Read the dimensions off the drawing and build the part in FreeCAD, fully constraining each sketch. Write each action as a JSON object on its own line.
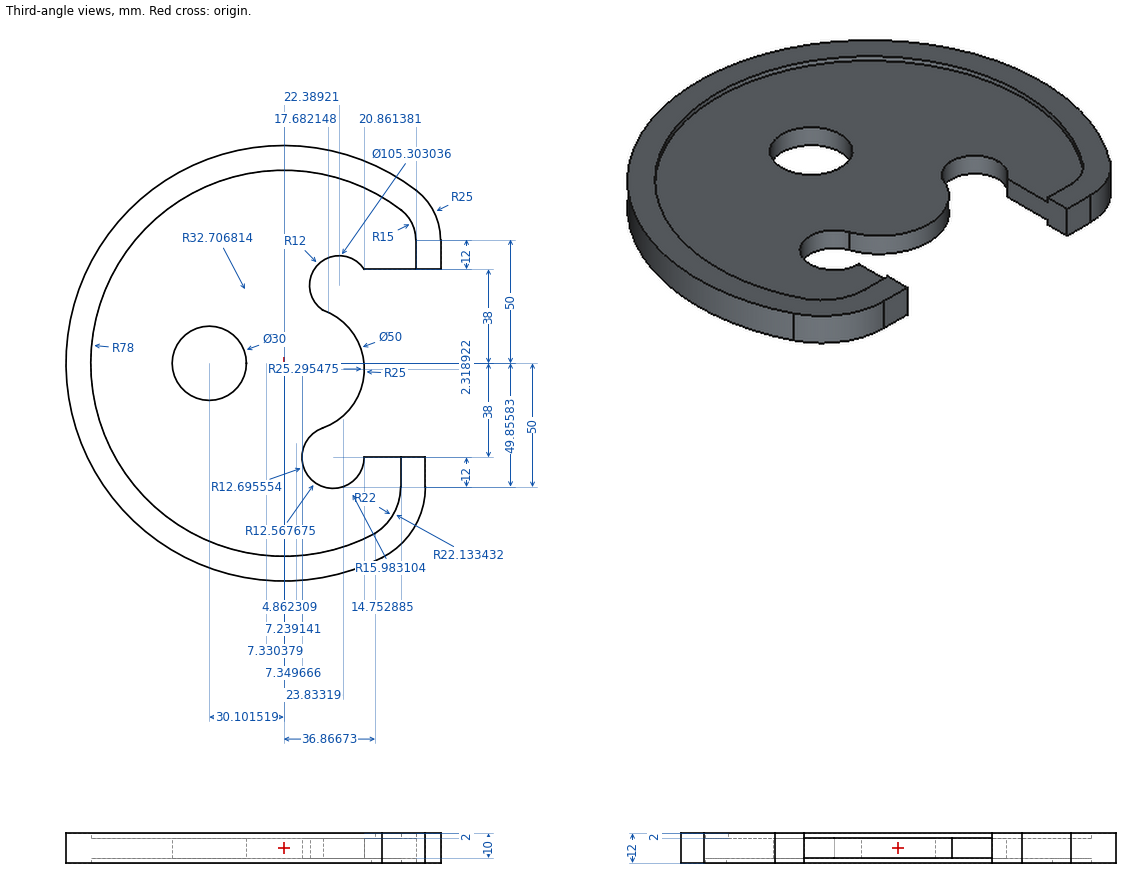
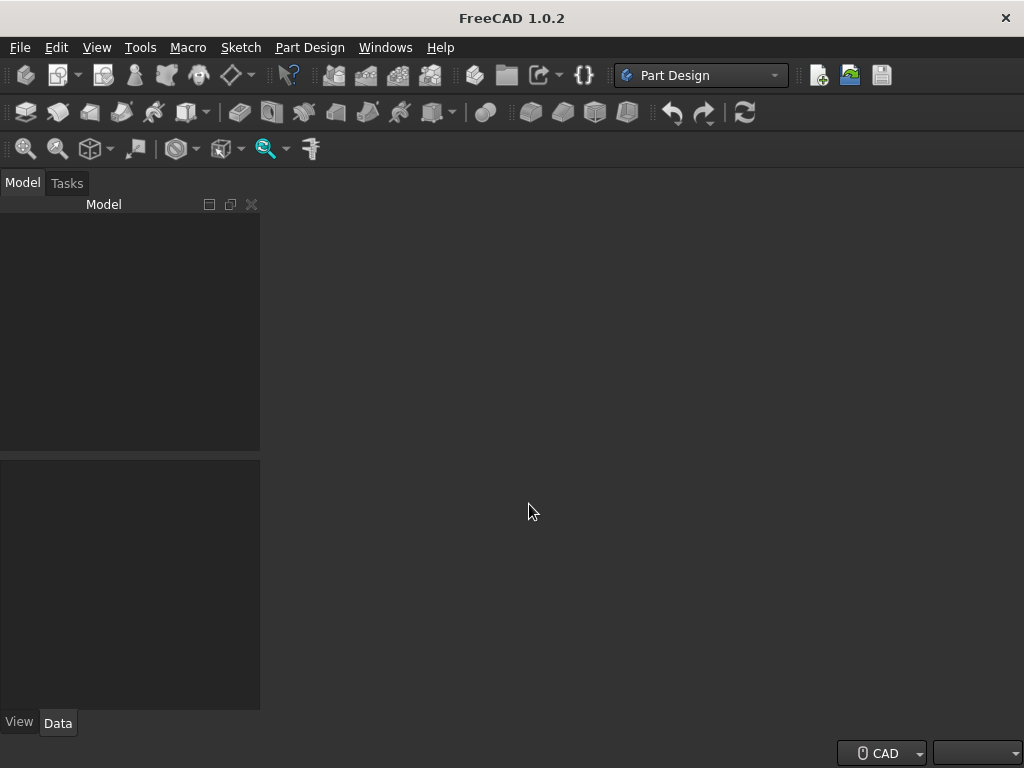
{"action": "key", "text": "ctrl+n"}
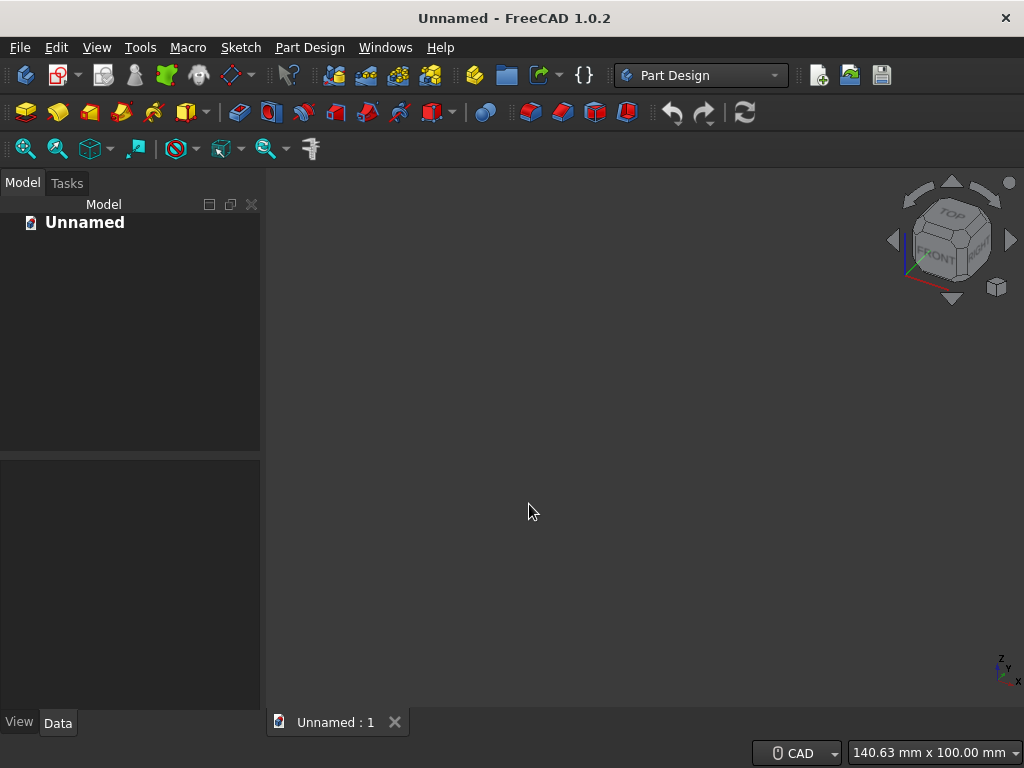
{"action": "left_click", "coordinate": [58, 76]}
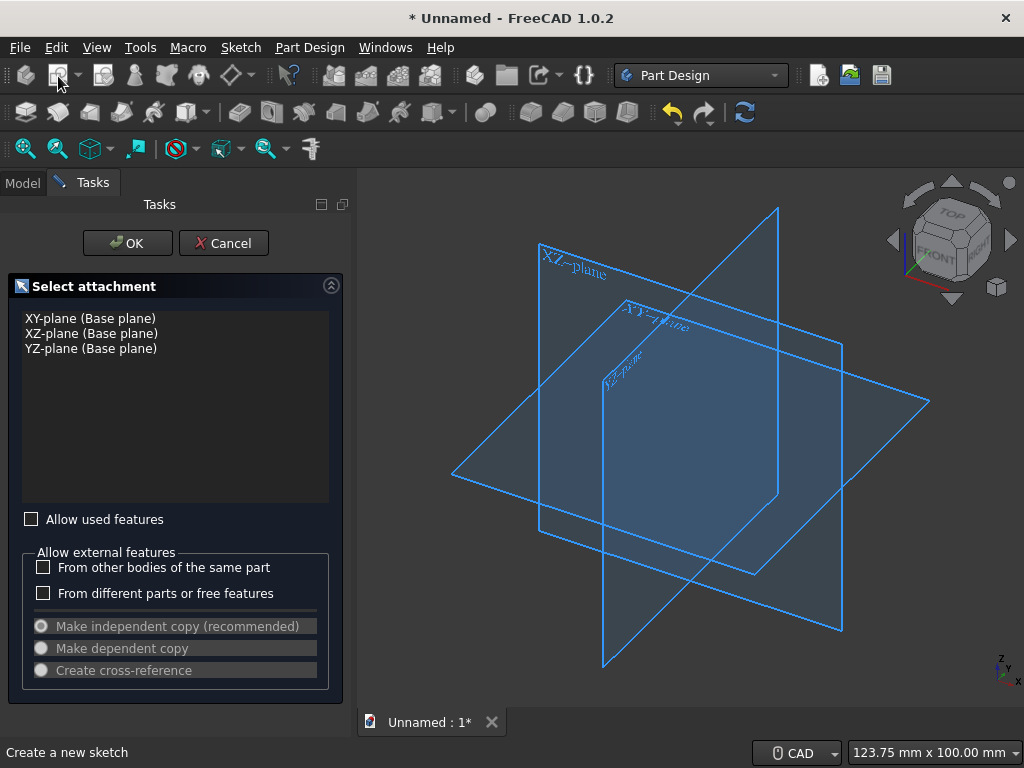
{"action": "left_click", "coordinate": [82, 318]}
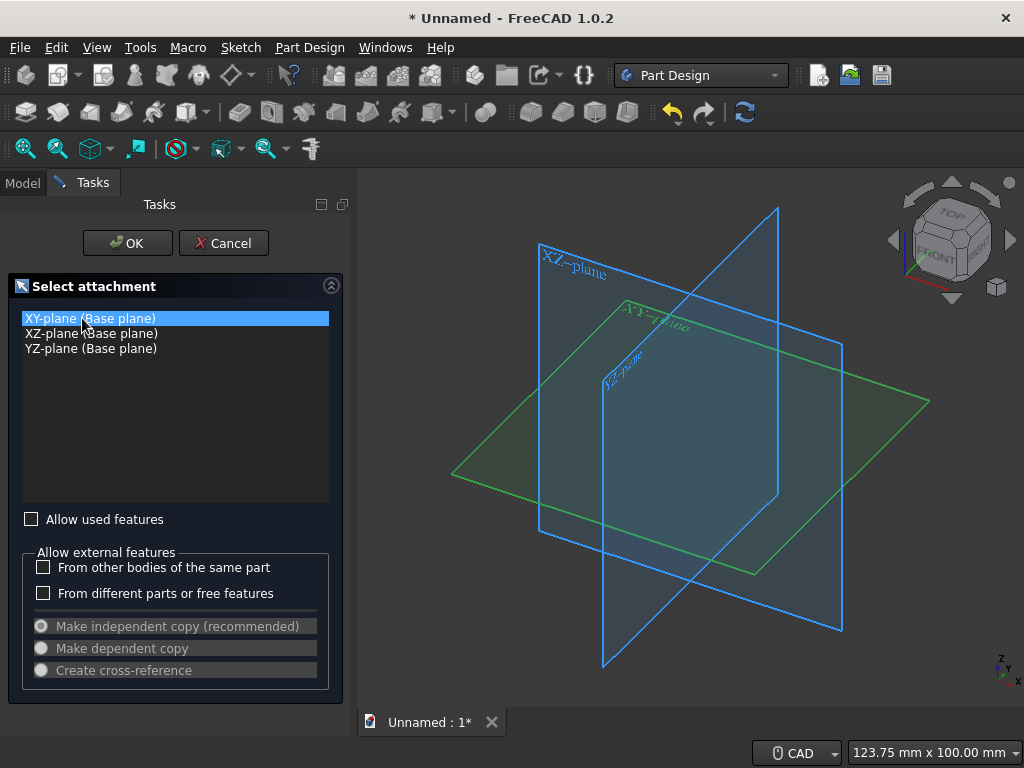
{"action": "left_click", "coordinate": [128, 243]}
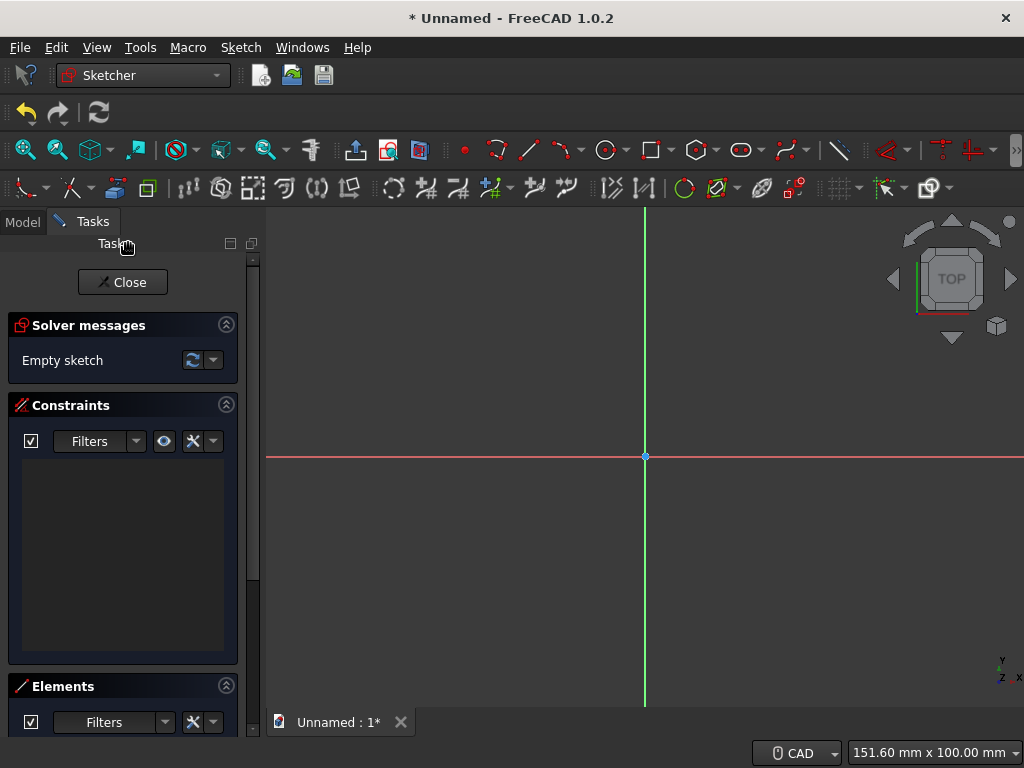
{"action": "scroll", "coordinate": [570, 439], "scroll_direction": "down", "scroll_amount": 4}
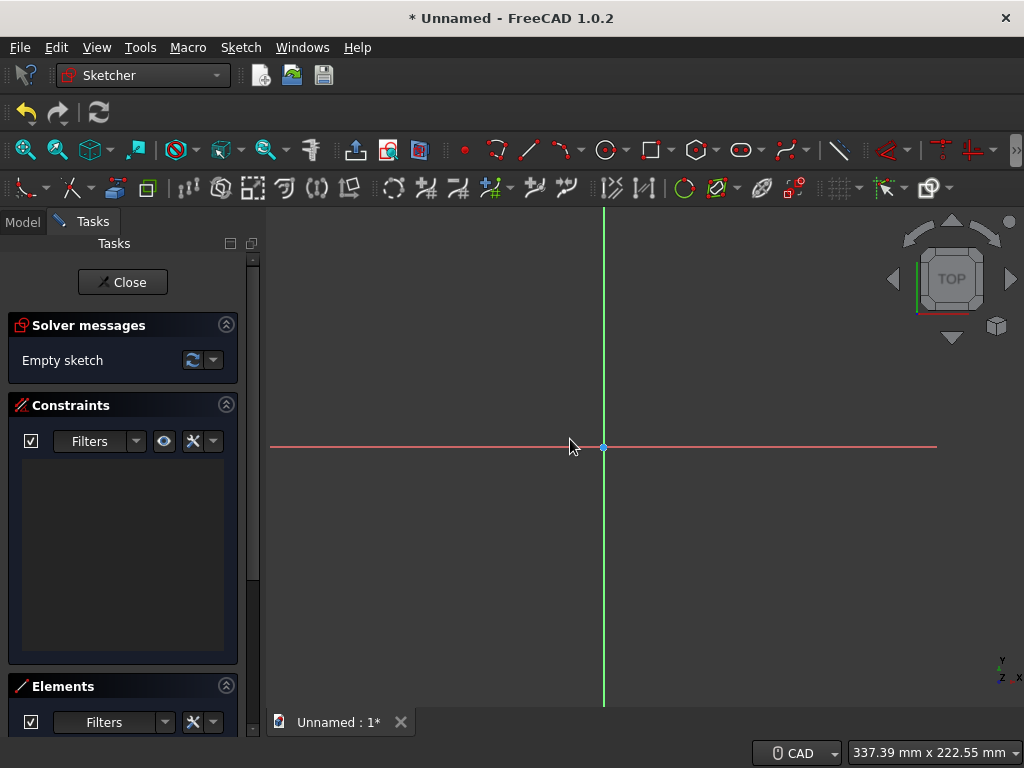
{"action": "key", "text": "g m"}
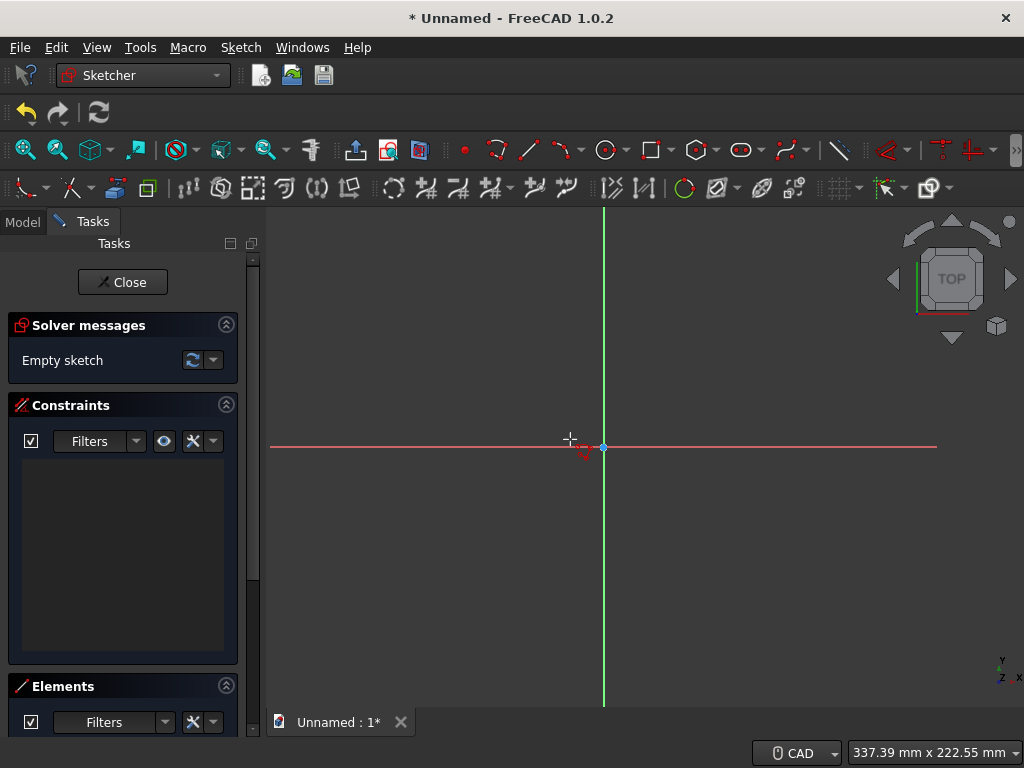
{"action": "left_click", "coordinate": [732, 560]}
{"action": "left_click", "coordinate": [732, 533]}
{"action": "left_click", "coordinate": [710, 533]}
{"action": "left_click", "coordinate": [710, 560]}
{"action": "right_click", "coordinate": [710, 560]}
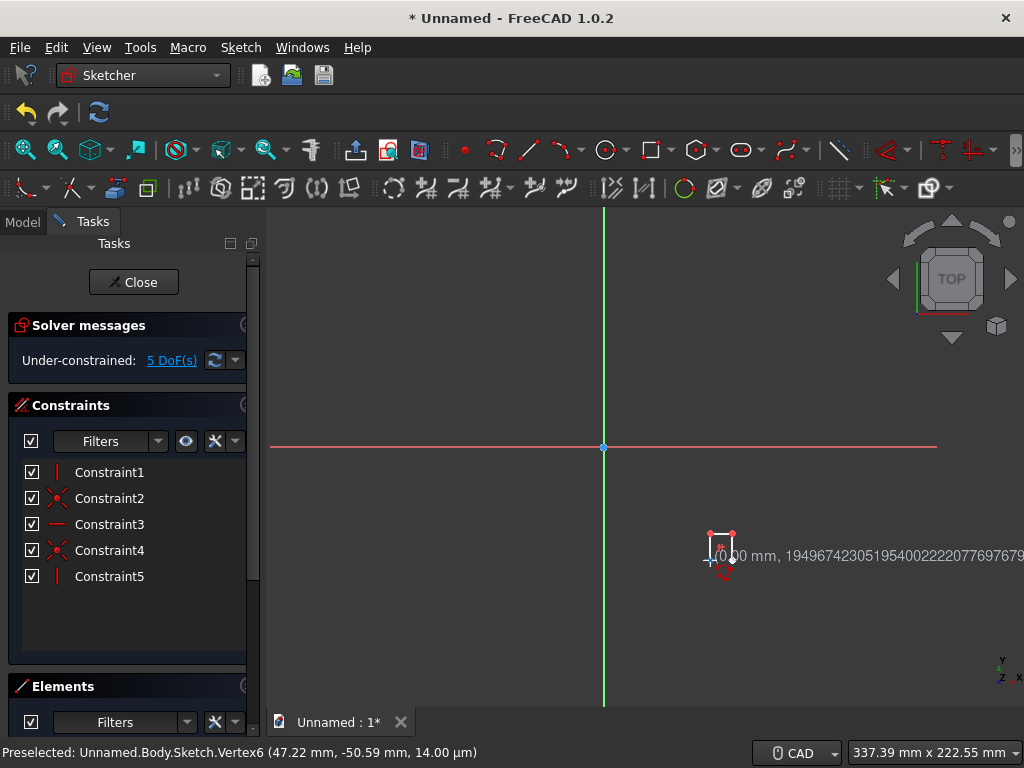
{"action": "left_click", "coordinate": [724, 335]}
{"action": "left_click", "coordinate": [724, 362]}
{"action": "left_click", "coordinate": [746, 362]}
{"action": "left_click", "coordinate": [746, 335]}
{"action": "right_click", "coordinate": [746, 335]}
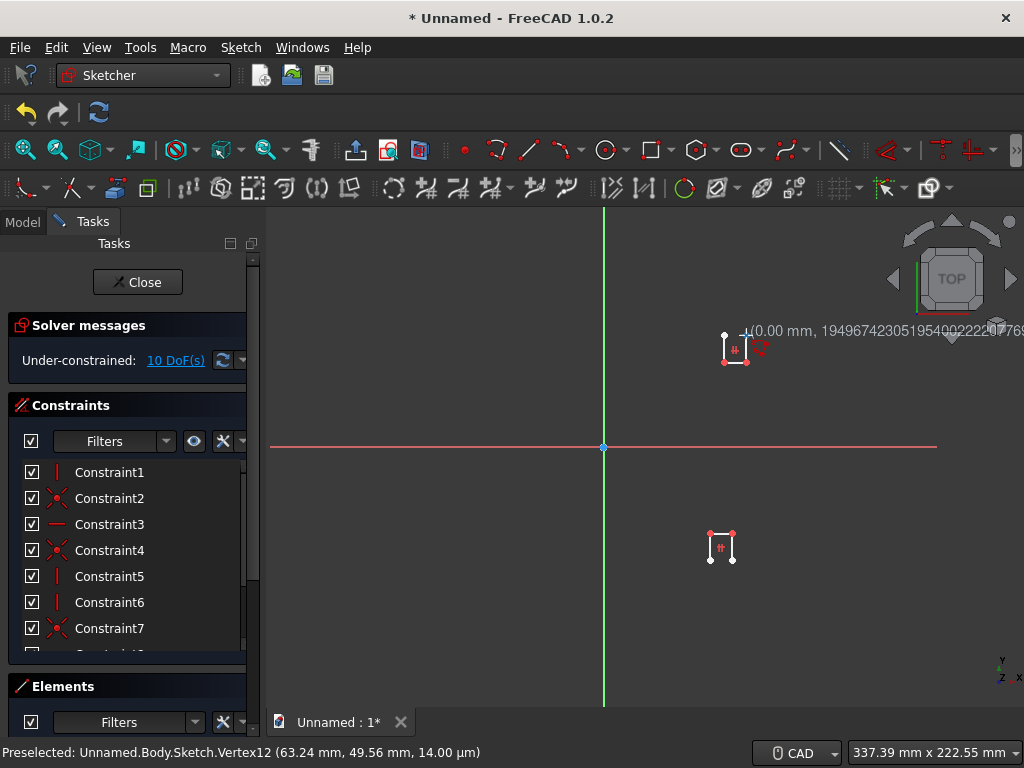
{"action": "key", "text": "g 3 a"}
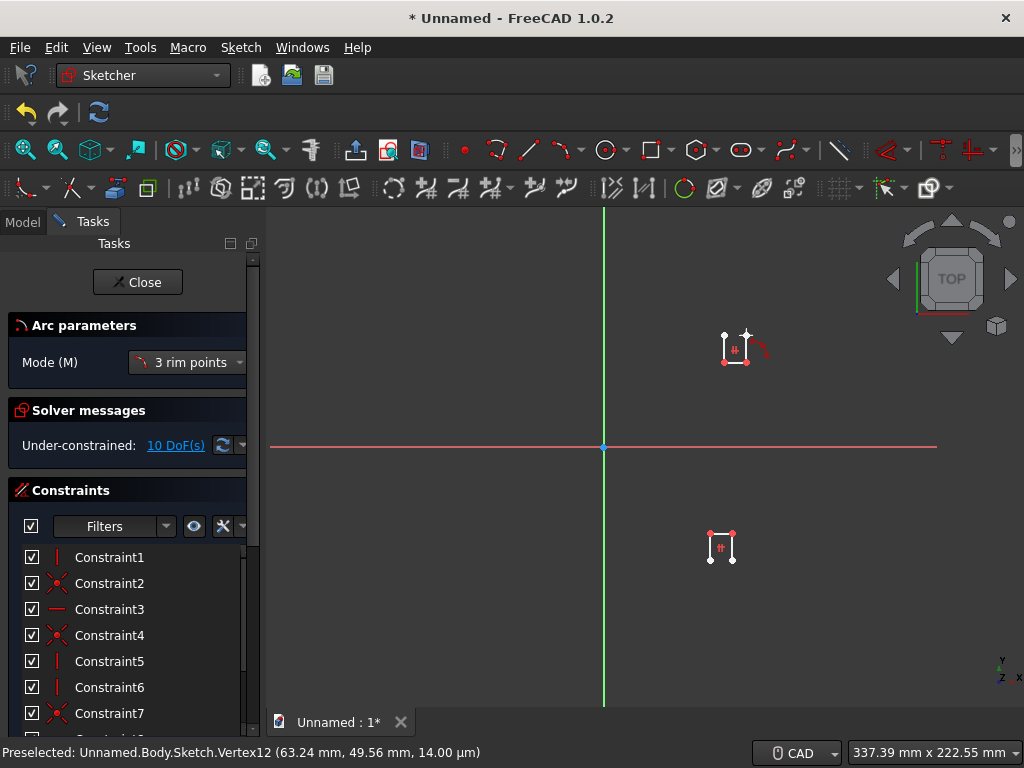
{"action": "left_click", "coordinate": [710, 561]}
{"action": "left_click", "coordinate": [683, 604]}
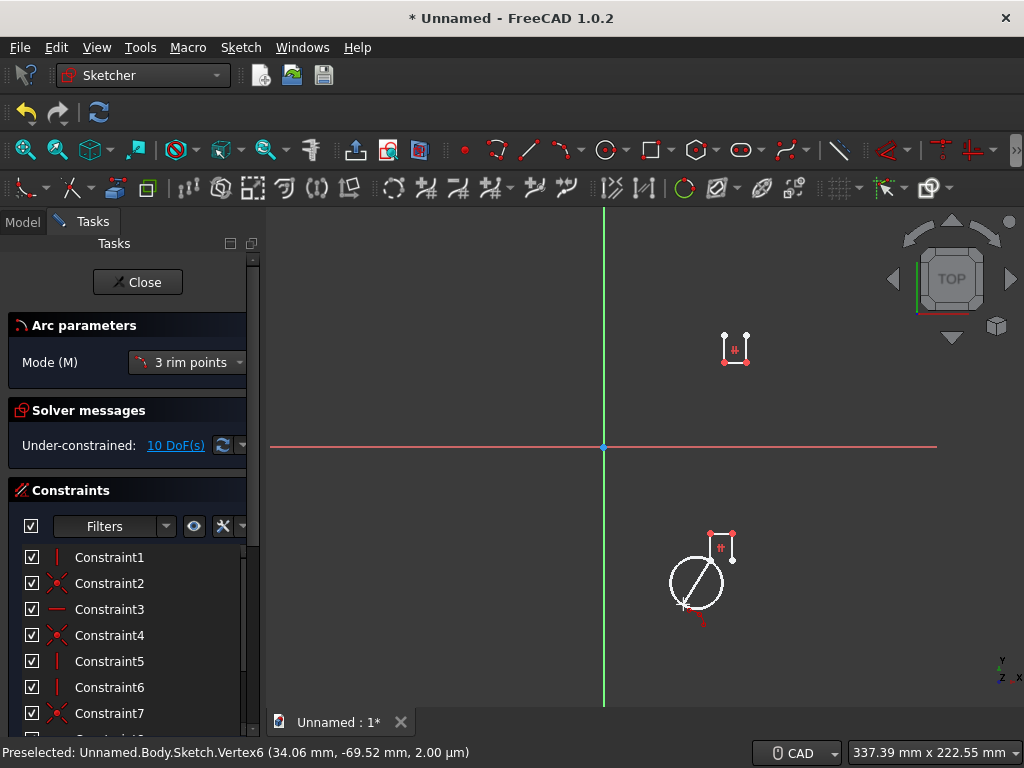
{"action": "scroll", "coordinate": [703, 586], "scroll_direction": "up", "scroll_amount": 4}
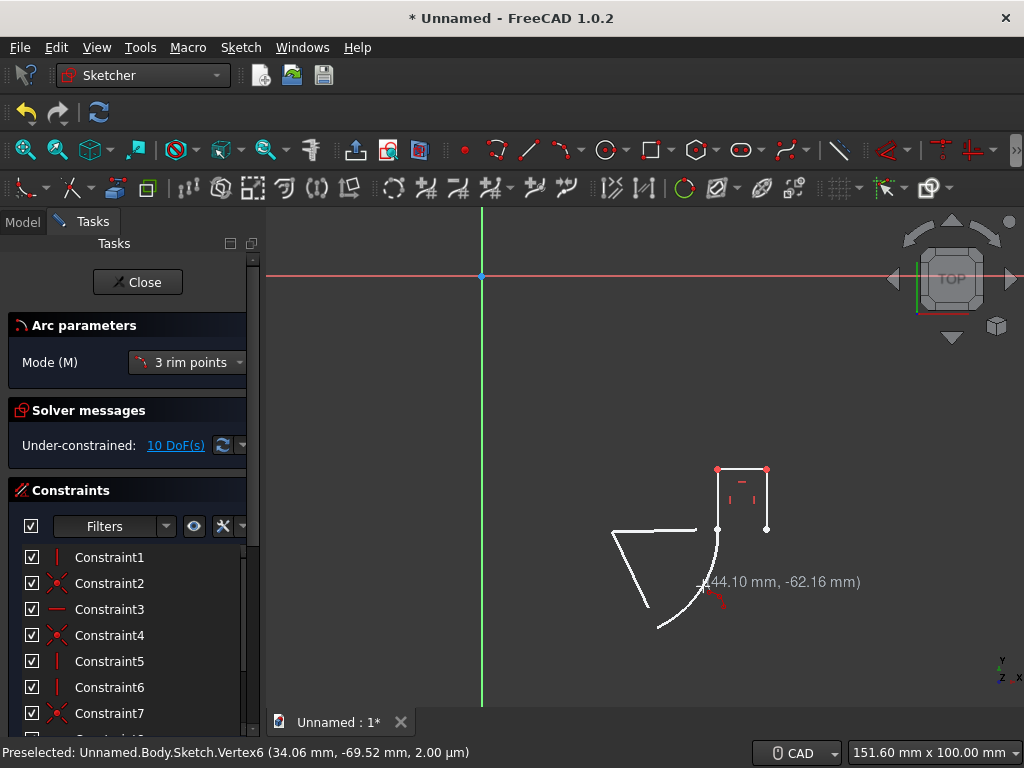
{"action": "left_click", "coordinate": [702, 584]}